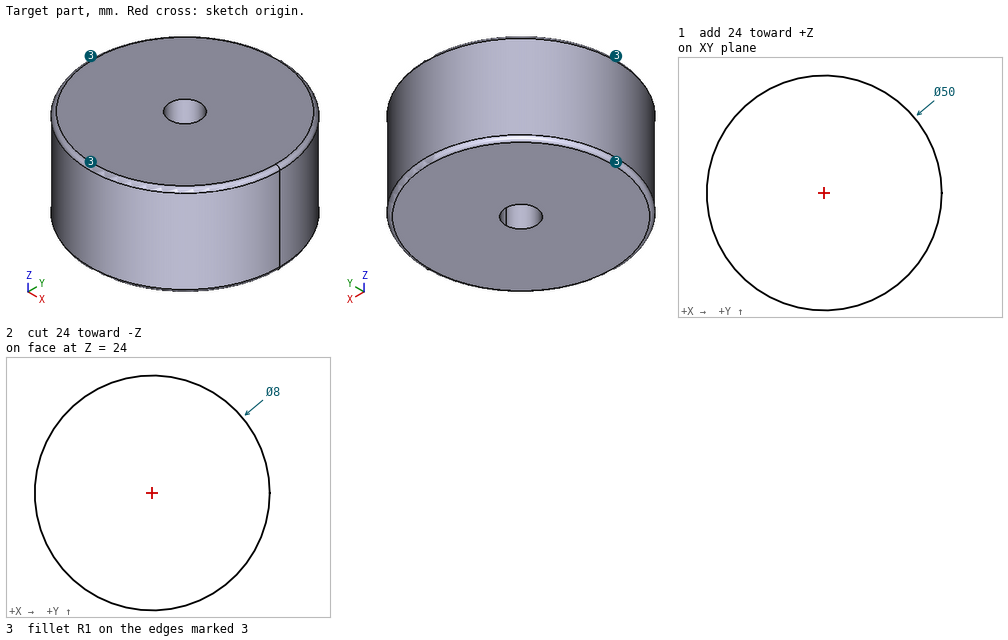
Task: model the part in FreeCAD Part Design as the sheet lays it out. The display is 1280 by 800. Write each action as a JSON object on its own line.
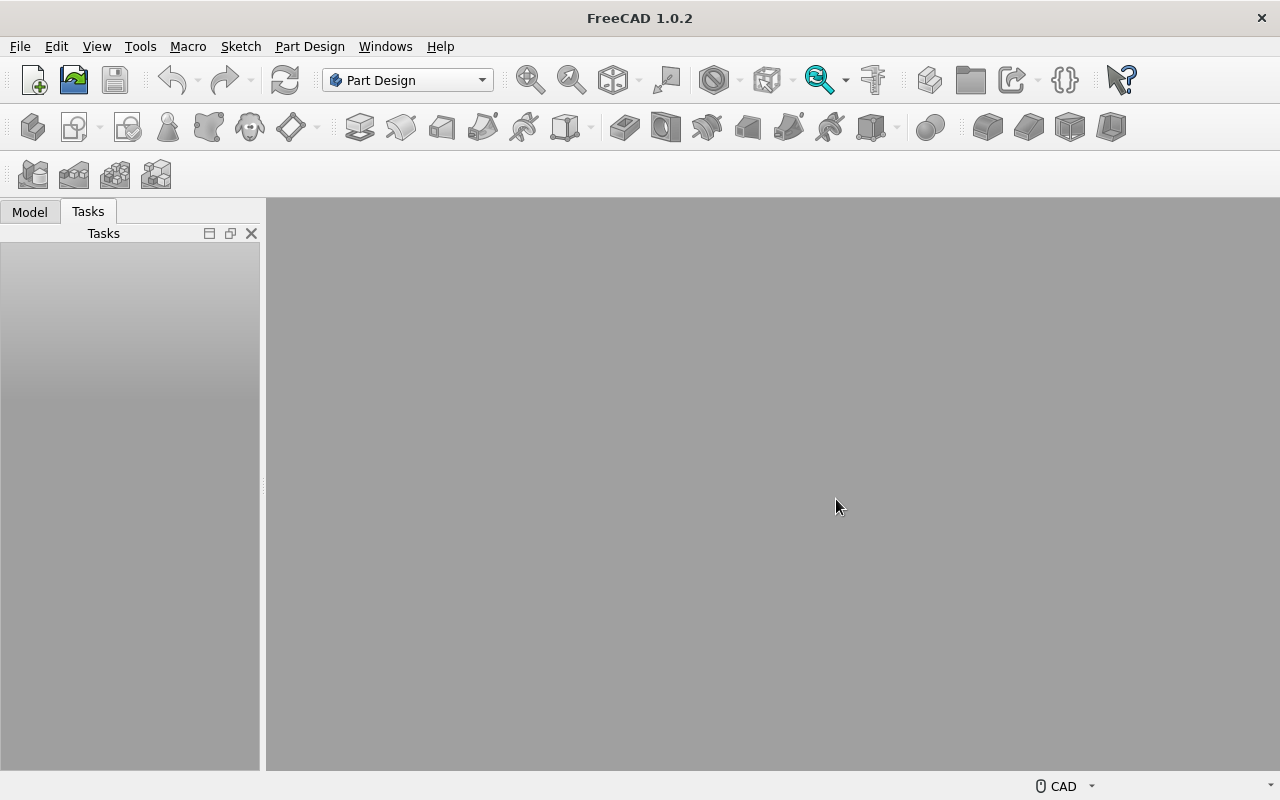
{"action": "left_click", "coordinate": [33, 80]}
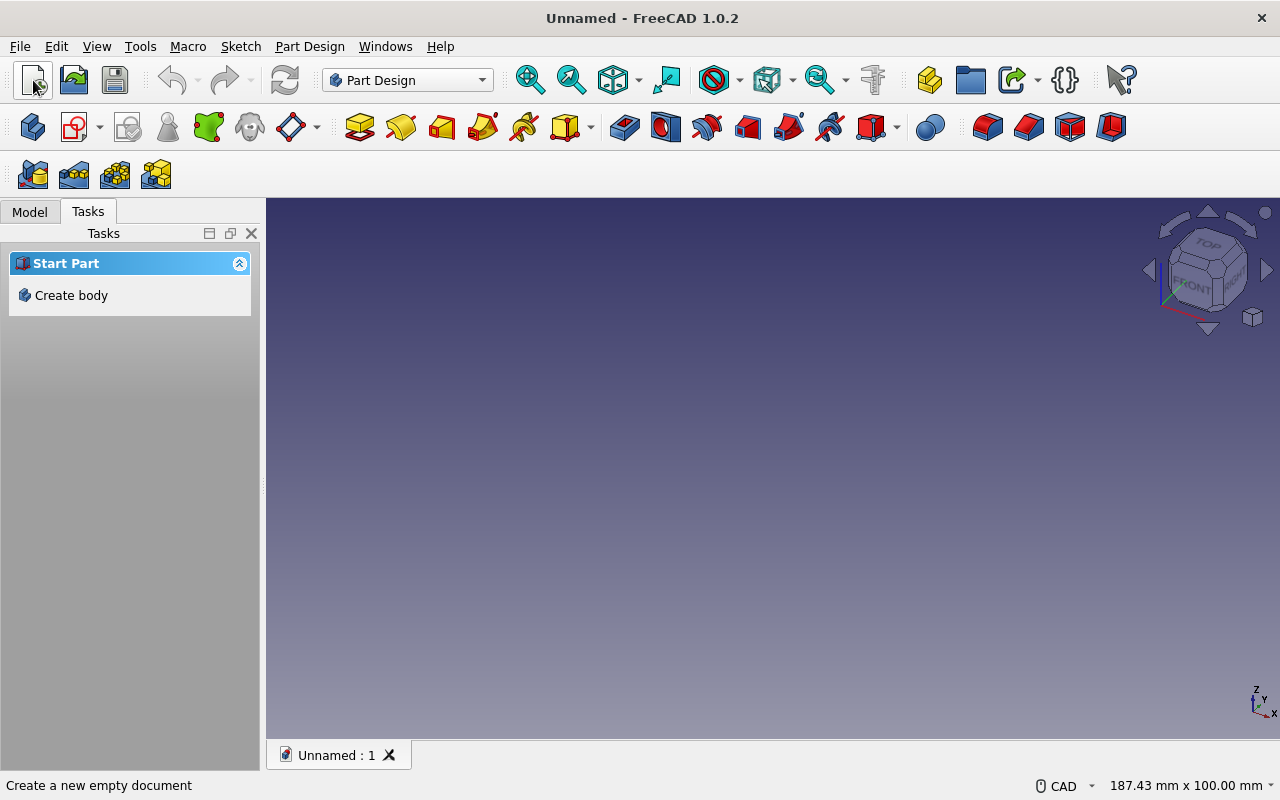
{"action": "left_click", "coordinate": [74, 128]}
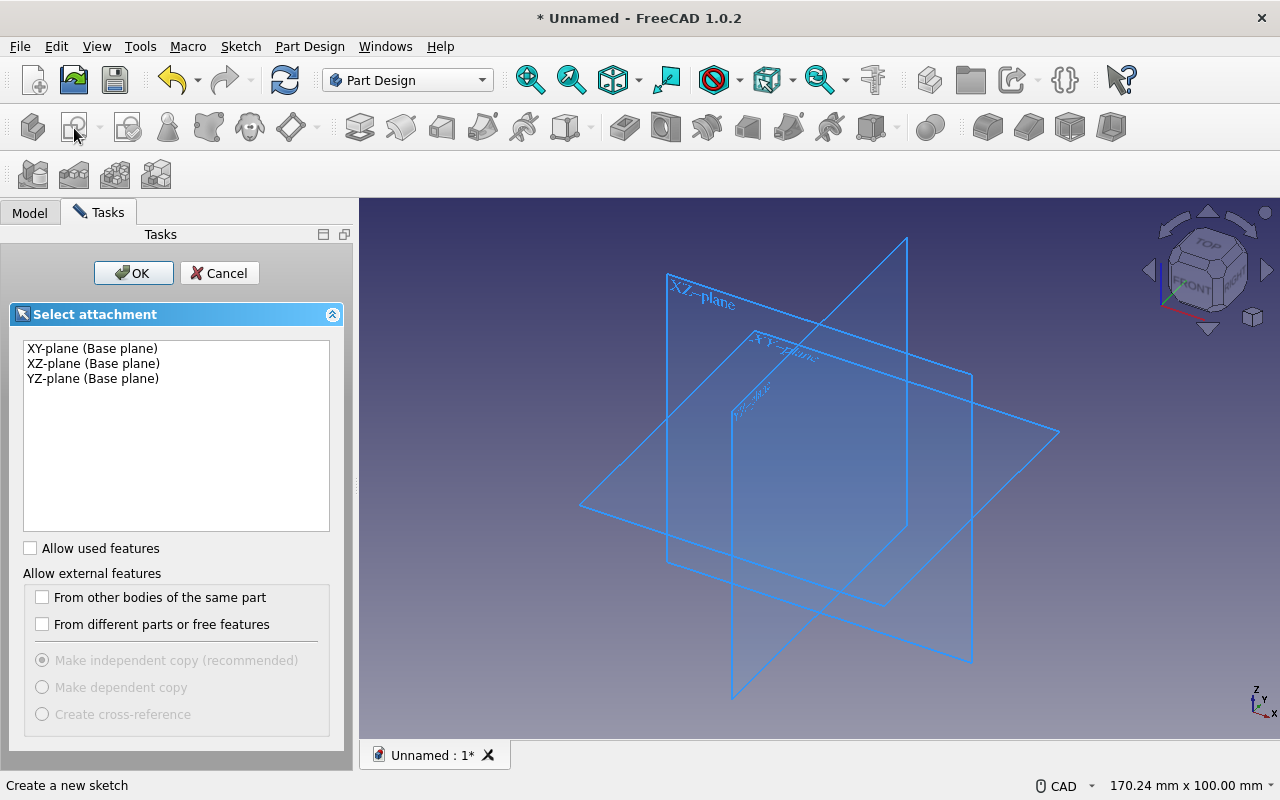
{"action": "left_click", "coordinate": [84, 348]}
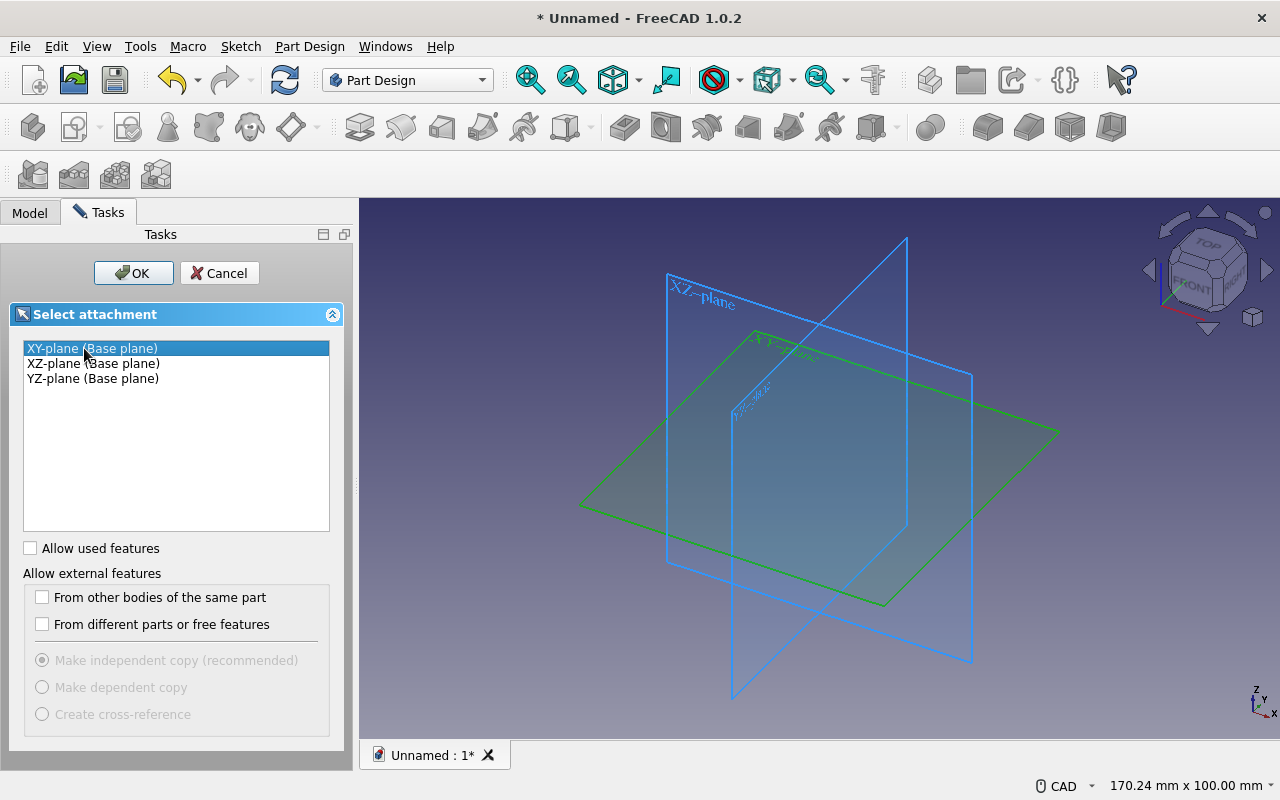
{"action": "left_click", "coordinate": [134, 273]}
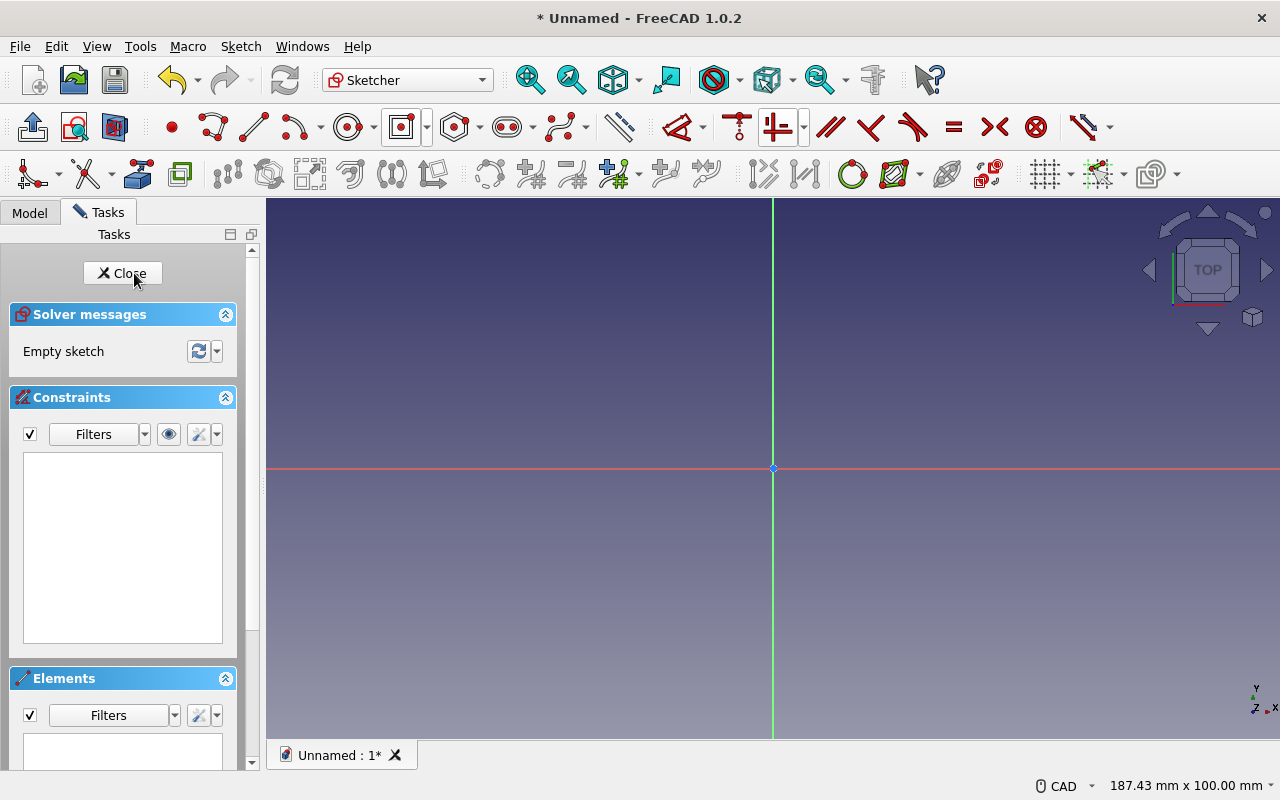
{"action": "left_click", "coordinate": [348, 128]}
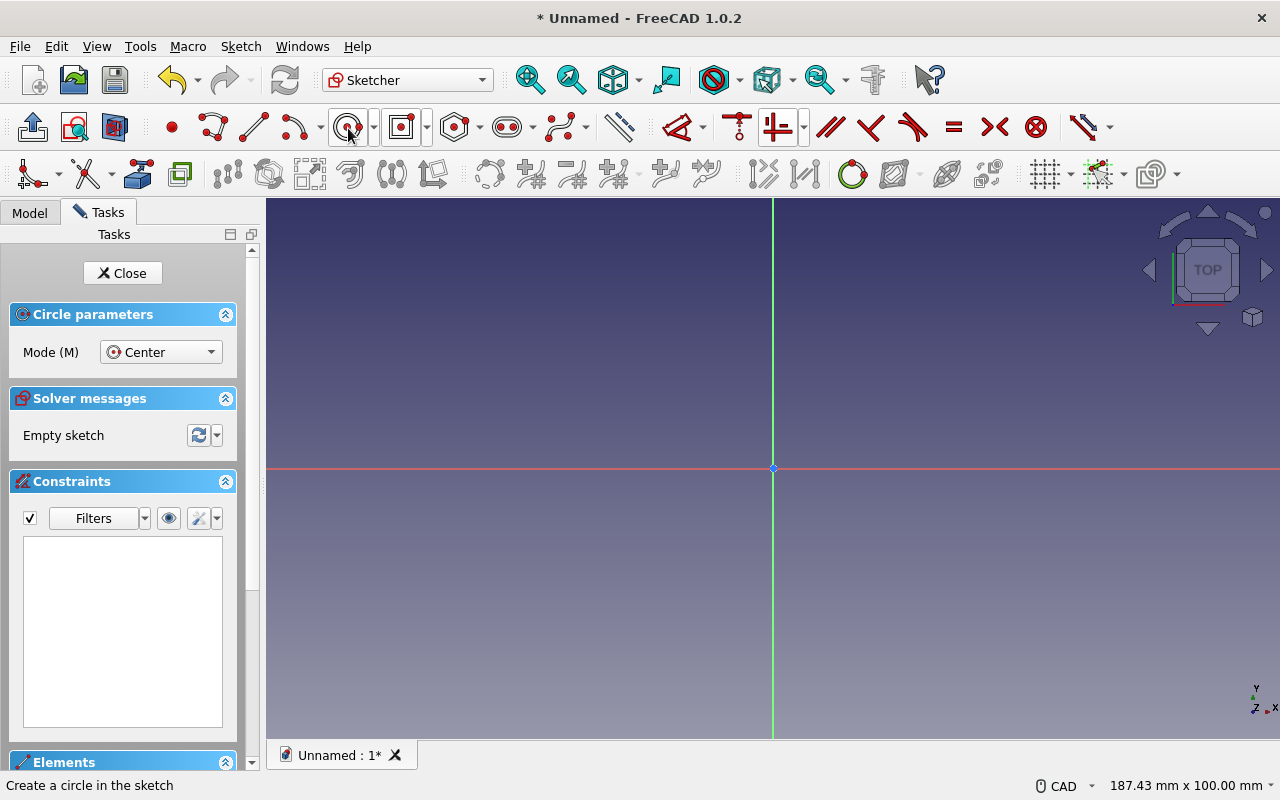
{"action": "left_click", "coordinate": [773, 468]}
{"action": "mouse_move", "coordinate": [869, 373]}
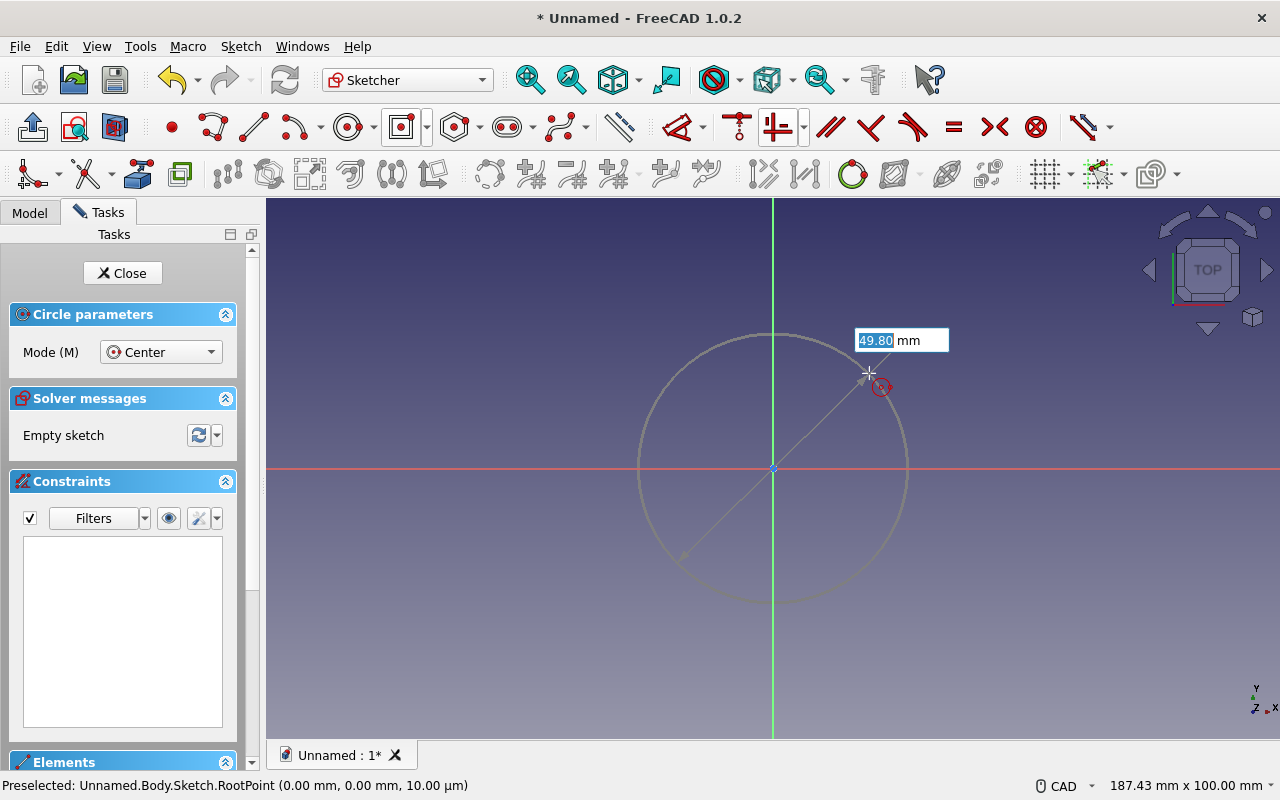
{"action": "type", "text": "50"}
{"action": "key", "text": "Return"}
{"action": "key", "text": "Escape"}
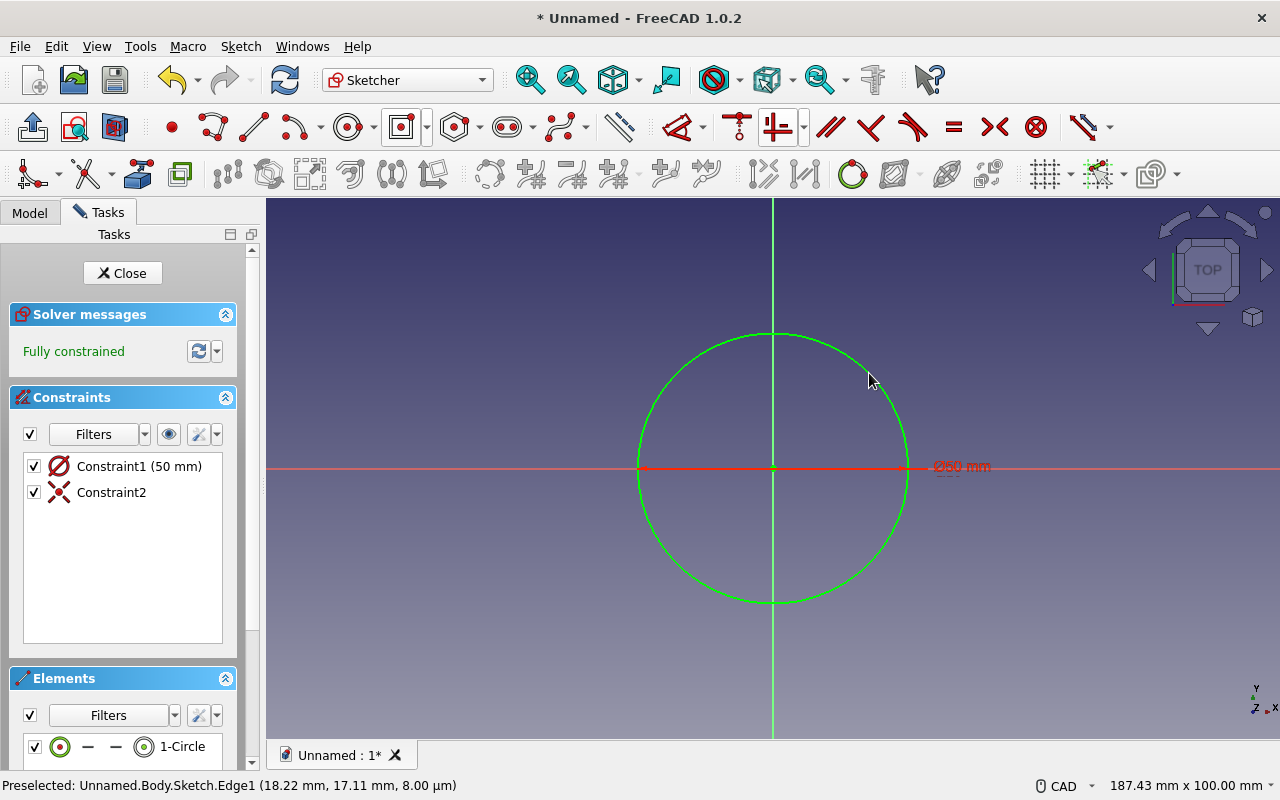
{"action": "left_click", "coordinate": [123, 273]}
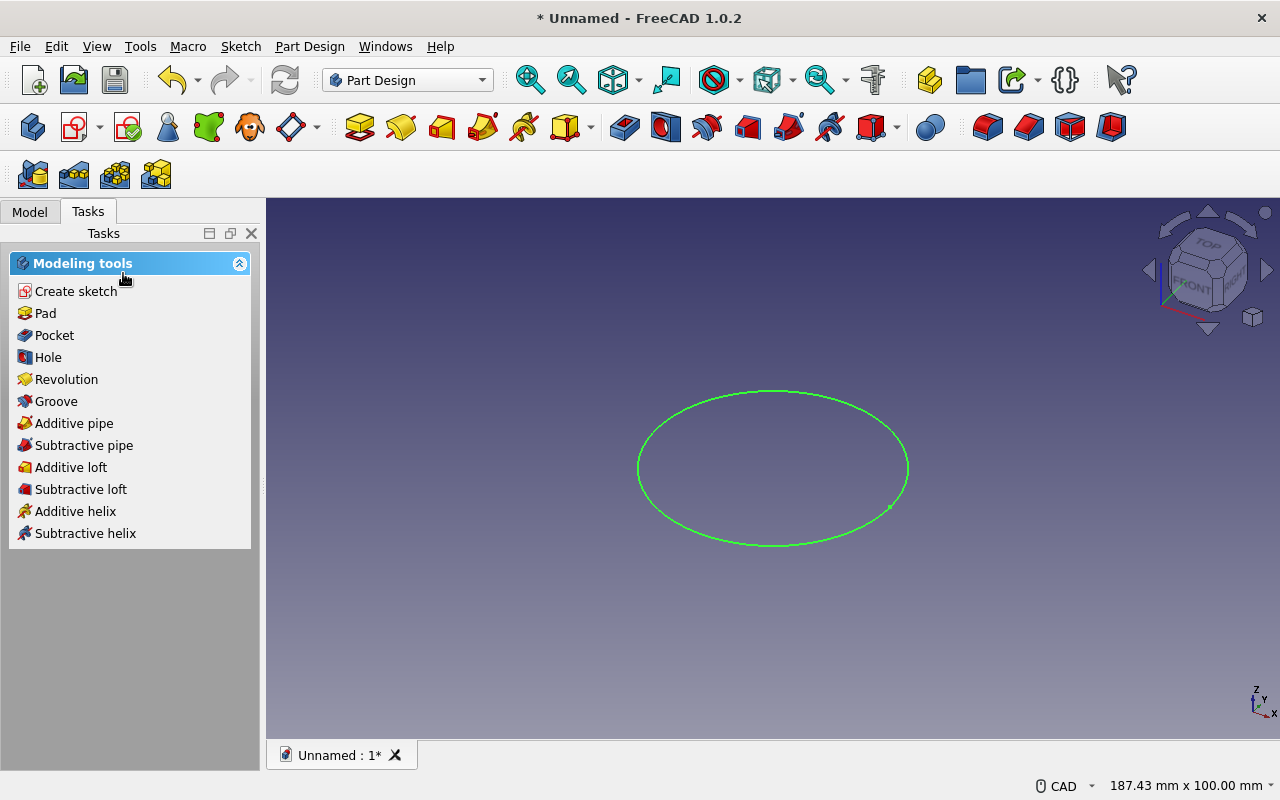
{"action": "left_click", "coordinate": [360, 128]}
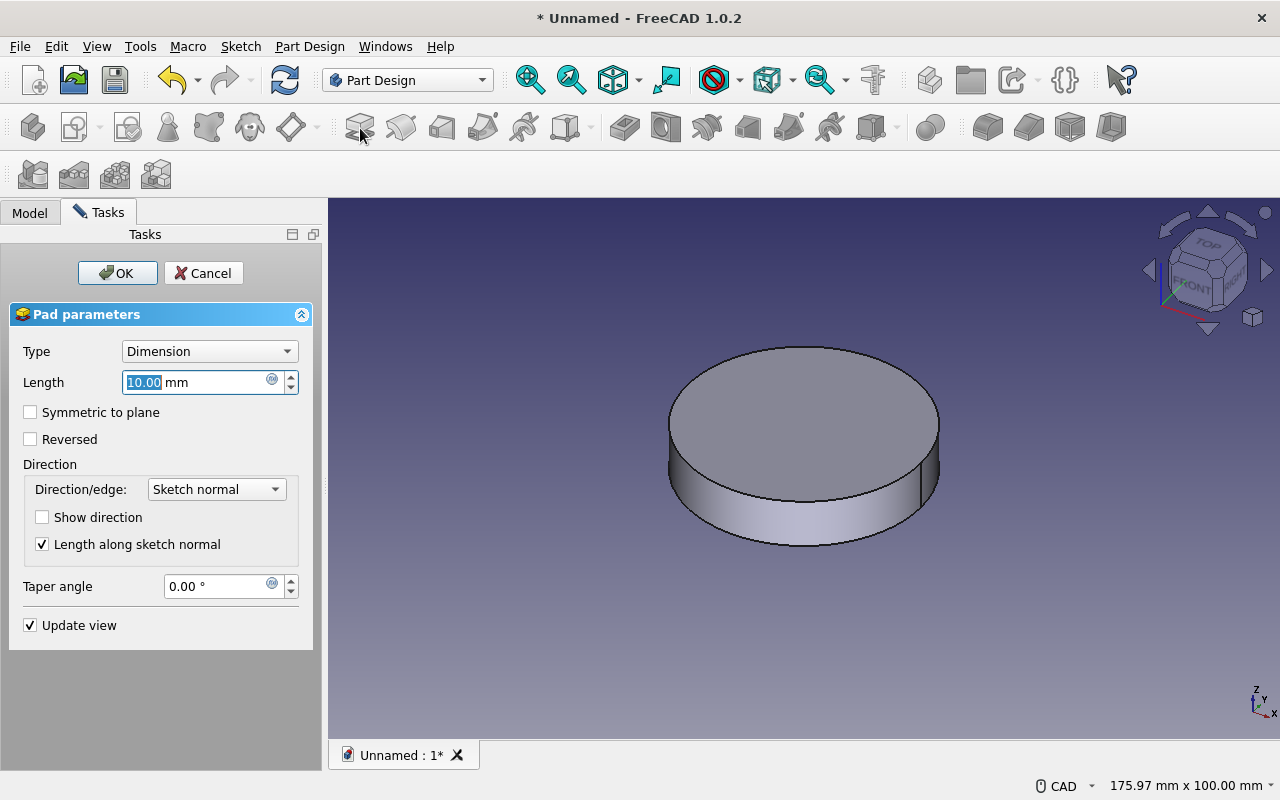
{"action": "type", "text": "24"}
{"action": "key", "text": "Tab"}